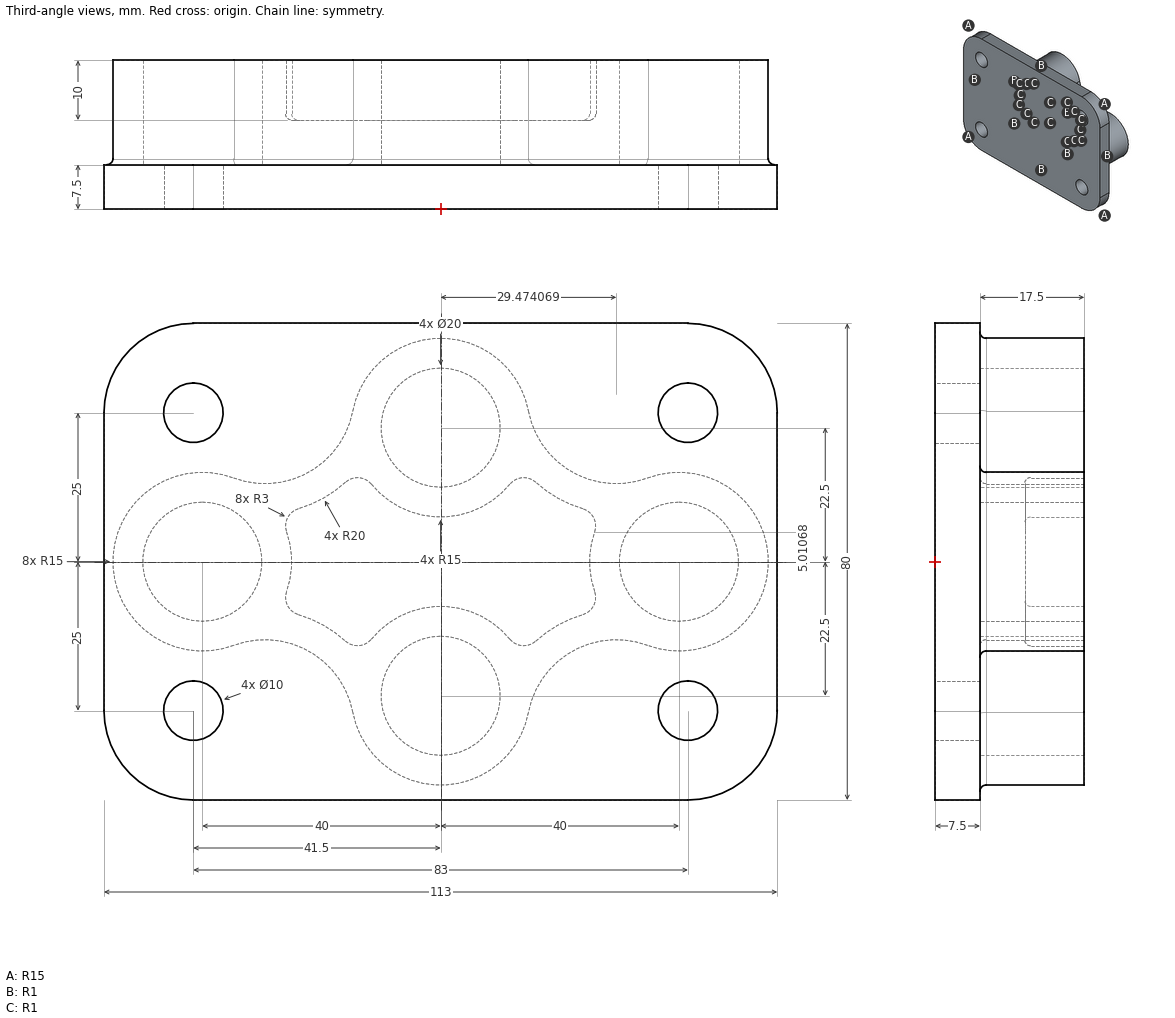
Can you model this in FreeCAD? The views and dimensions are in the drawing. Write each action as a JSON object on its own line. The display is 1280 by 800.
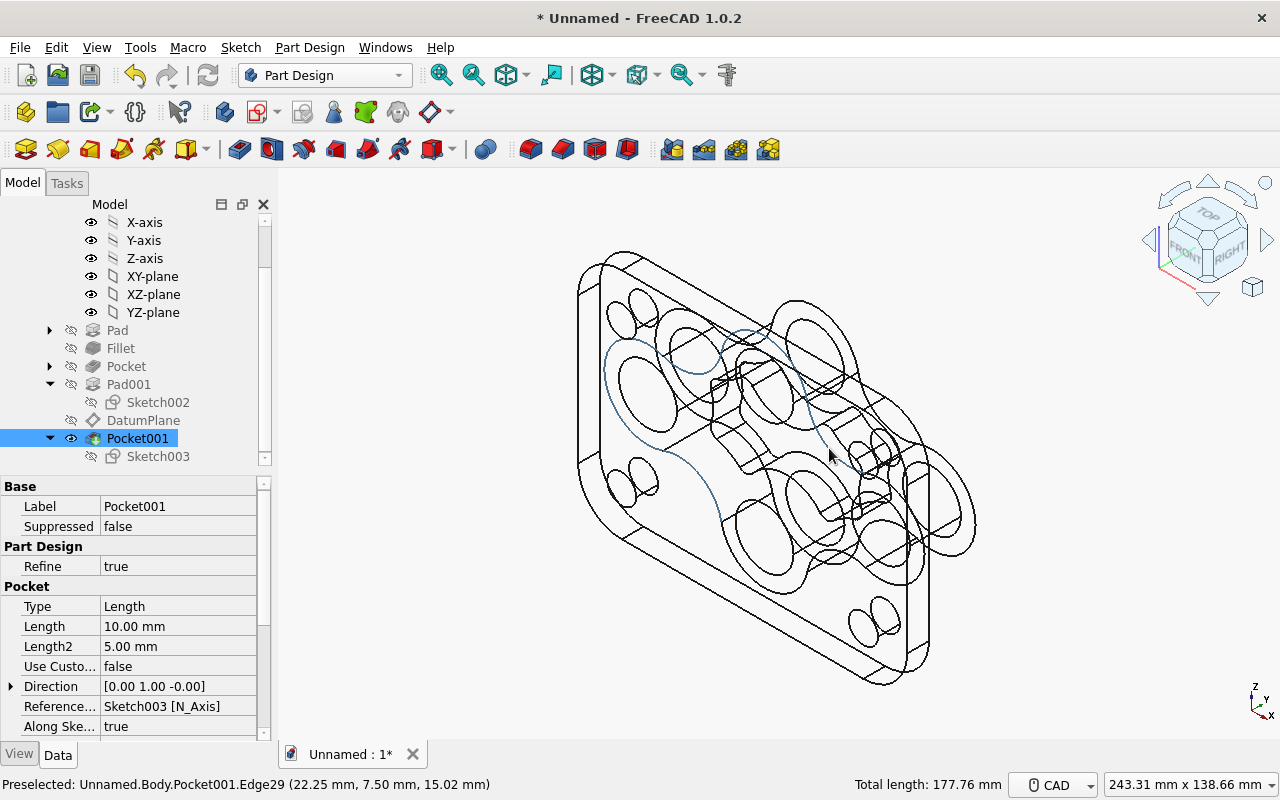
{"action": "left_click", "coordinate": [921, 533], "text": "ctrl"}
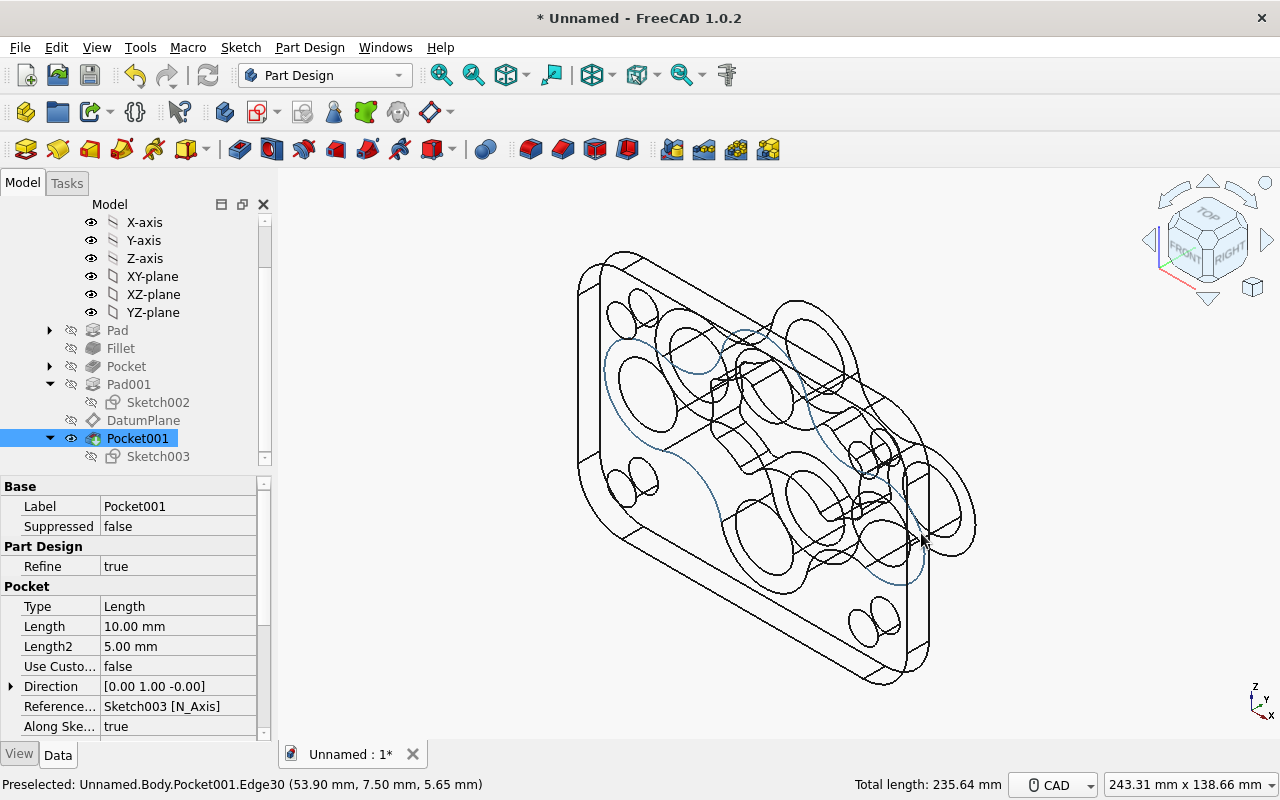
{"action": "left_click", "coordinate": [829, 549], "text": "ctrl"}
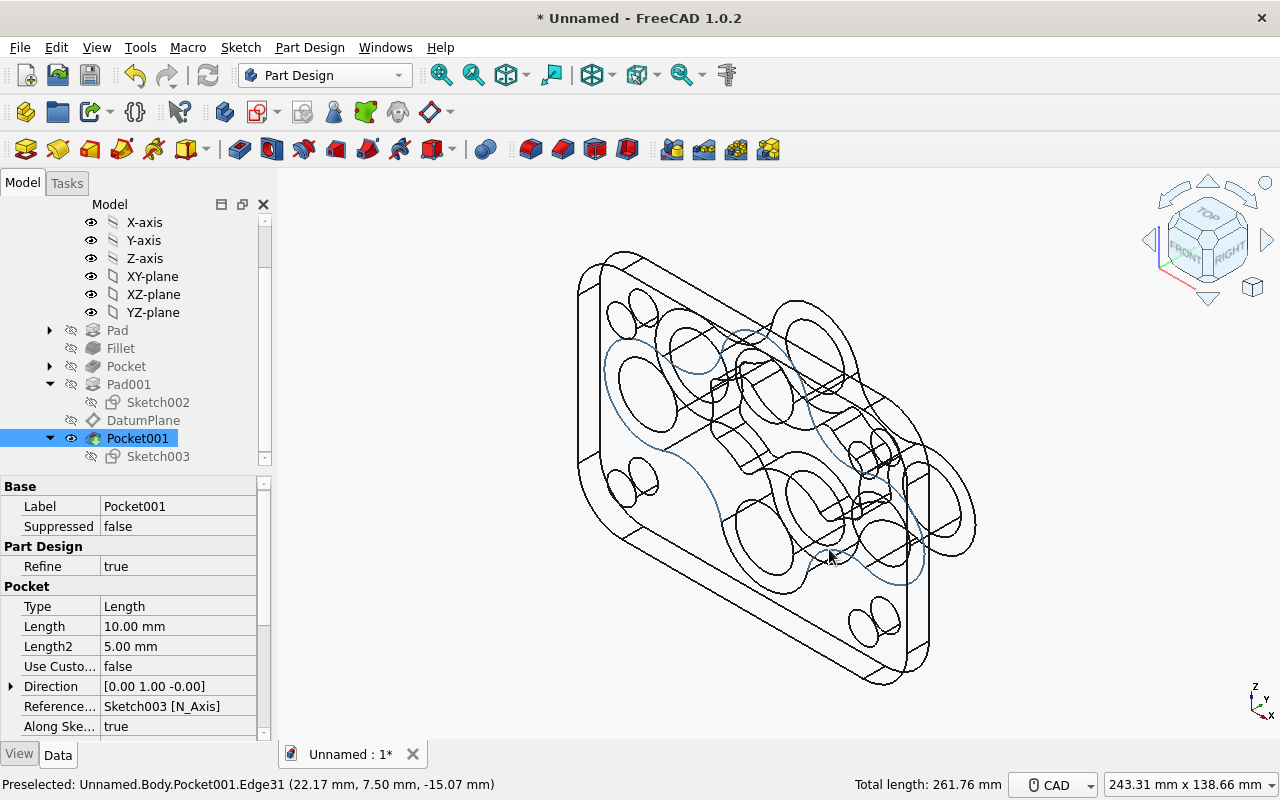
{"action": "left_click", "coordinate": [764, 587], "text": "ctrl"}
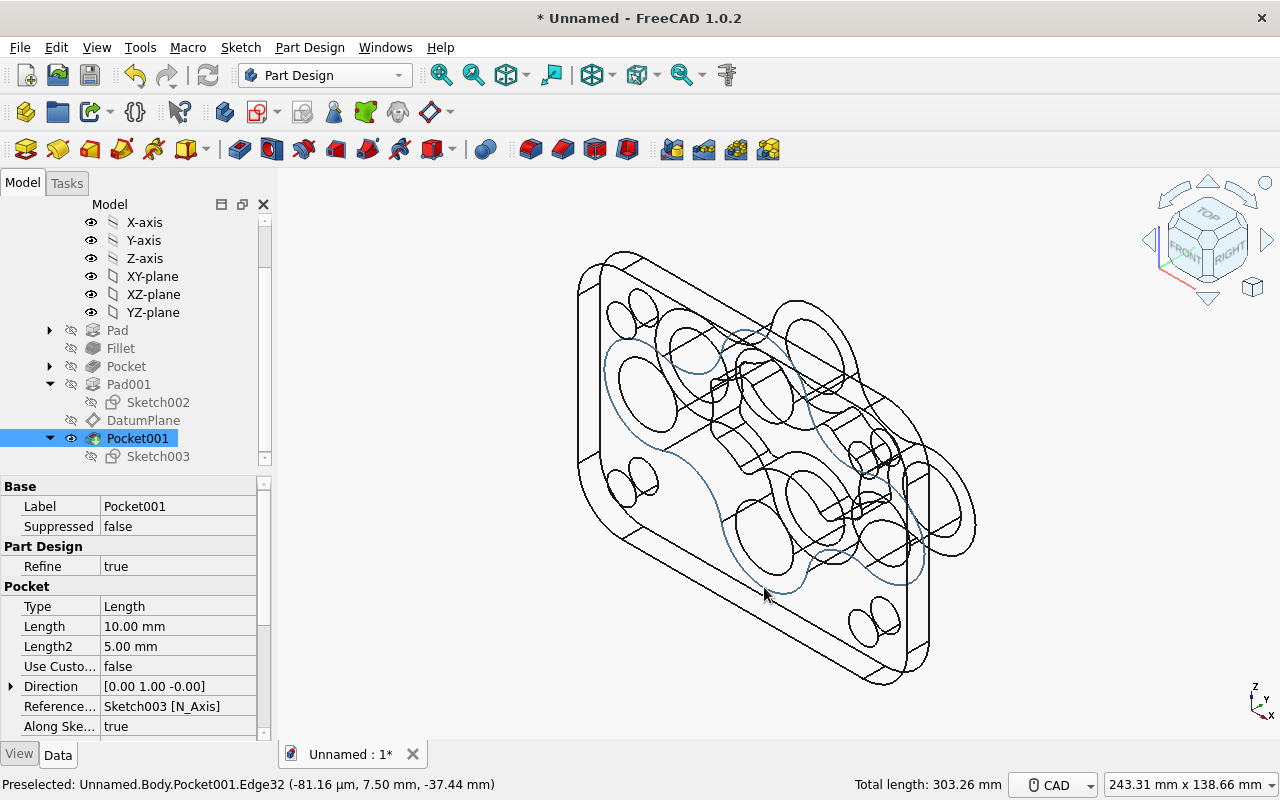
{"action": "key", "text": "v 1"}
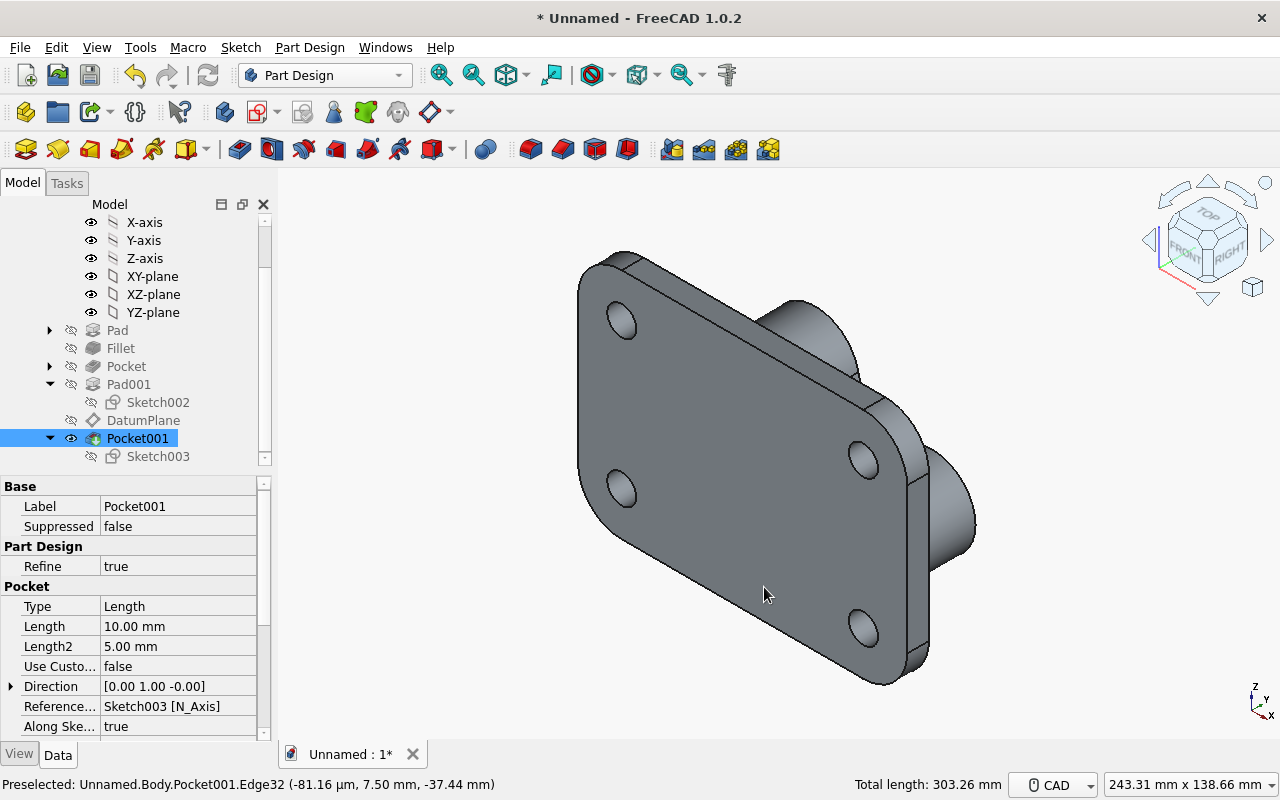
{"action": "left_click", "coordinate": [532, 150]}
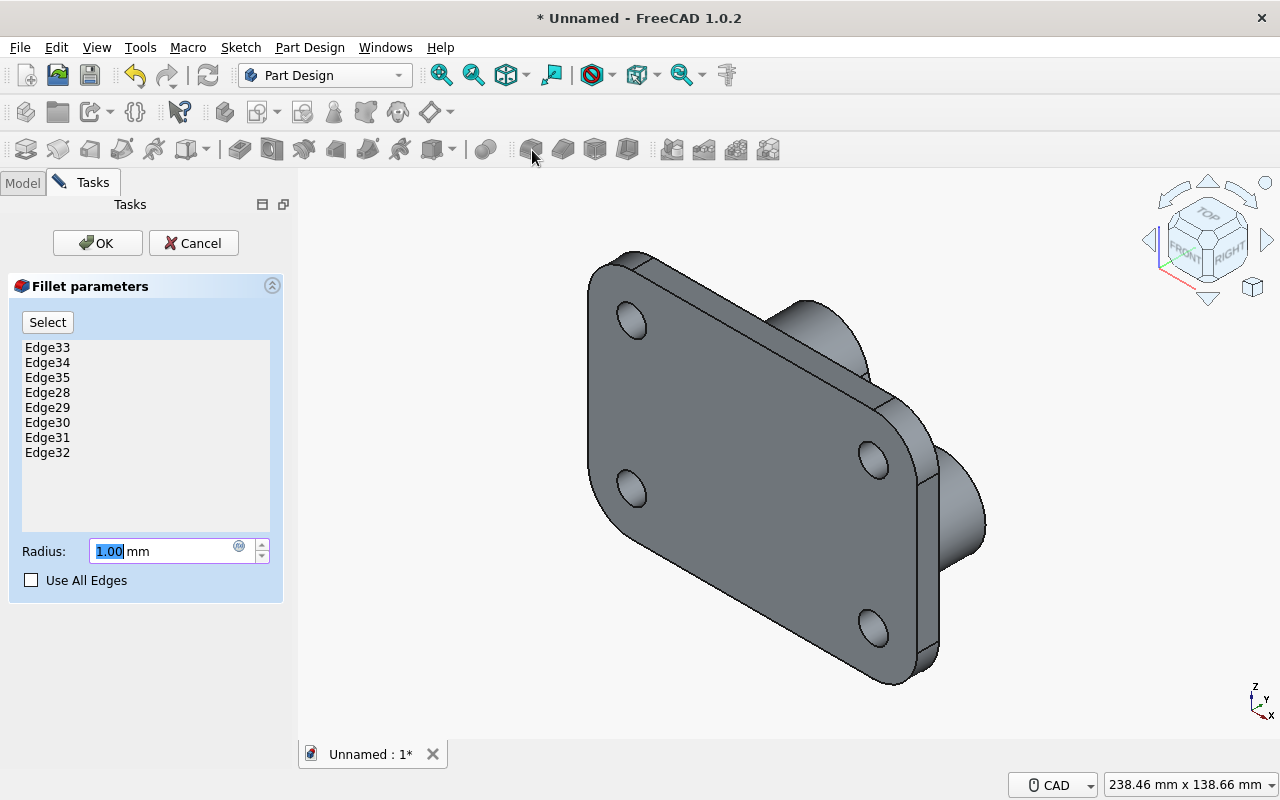
{"action": "type", "text": "1"}
{"action": "key", "text": "Tab"}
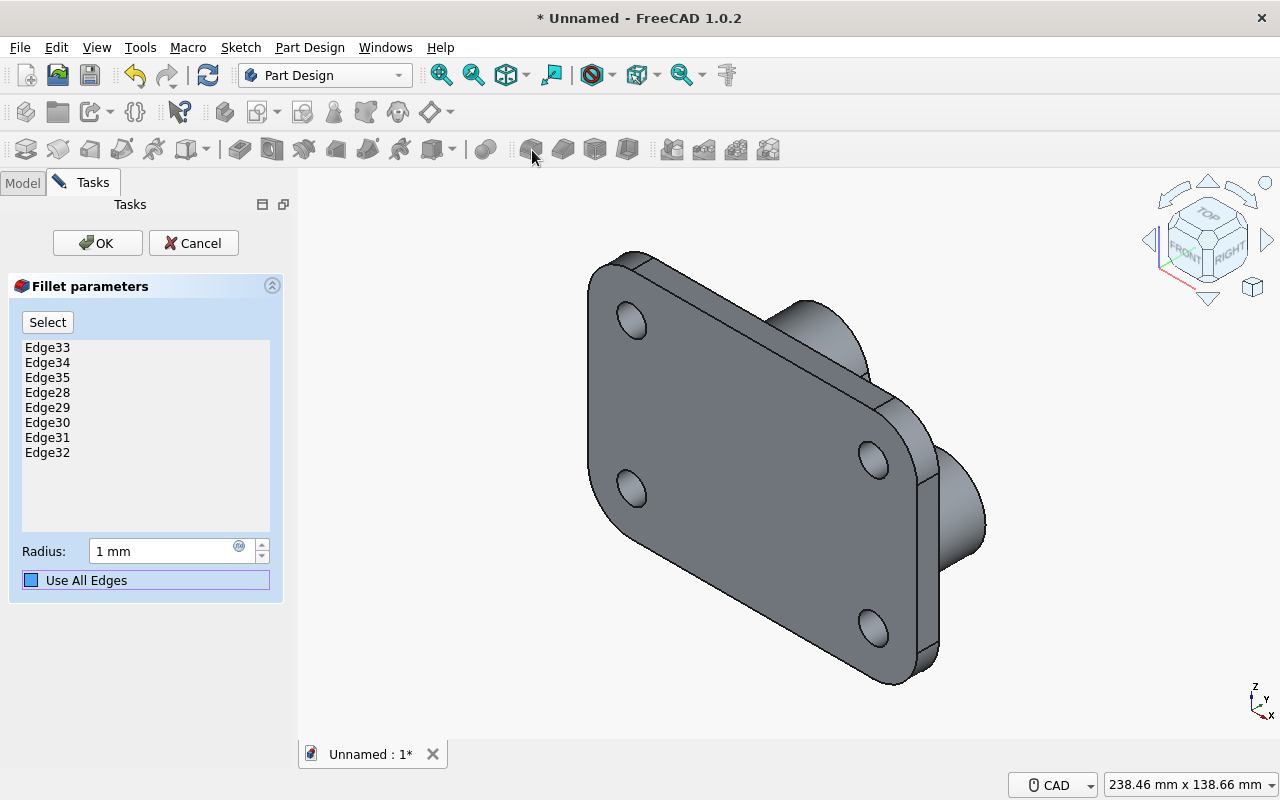
{"action": "left_click", "coordinate": [98, 243]}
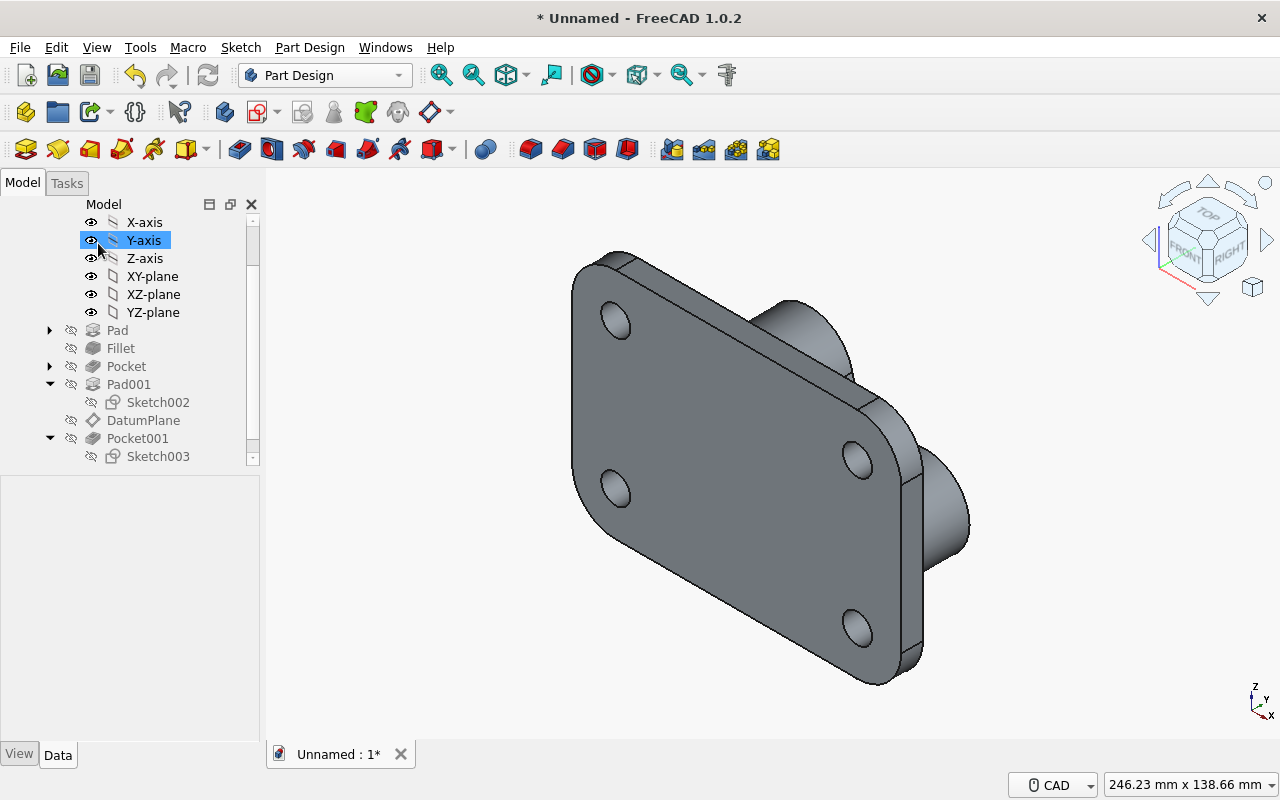
{"action": "key", "text": "2"}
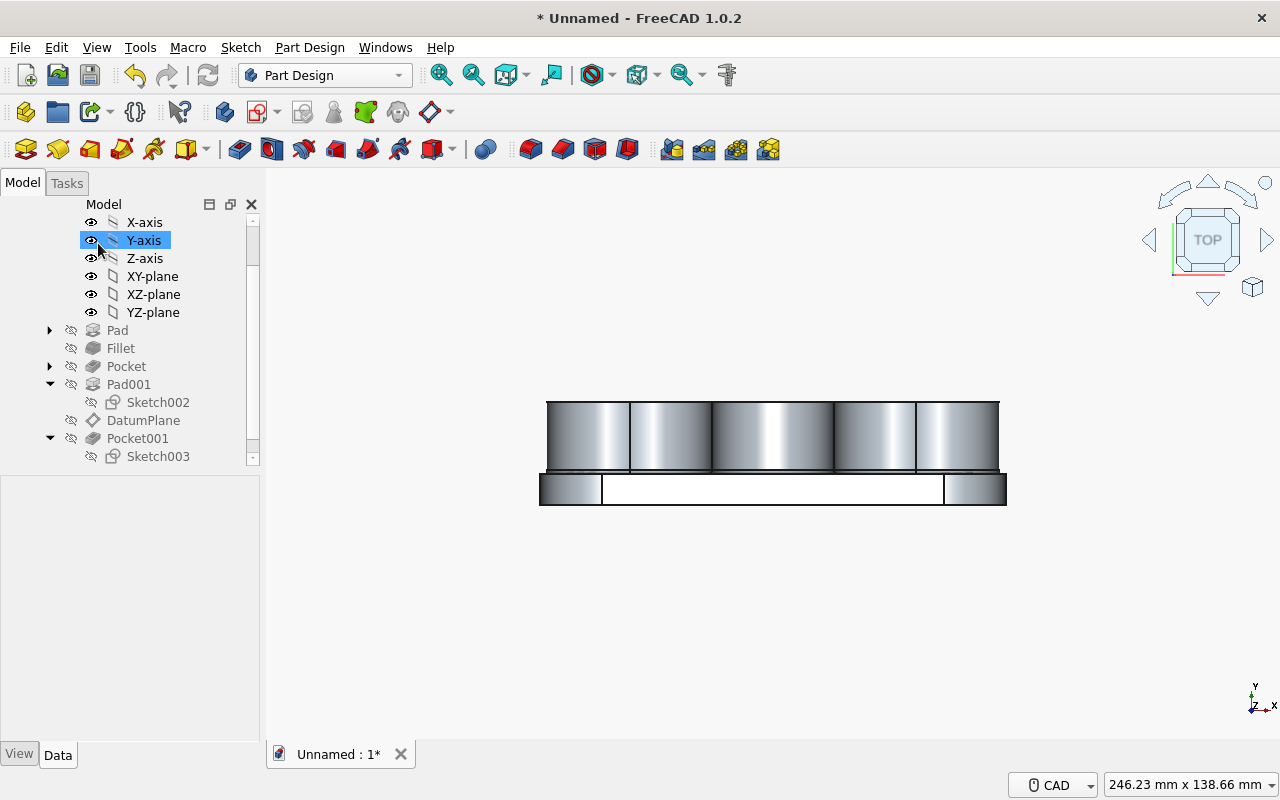
{"action": "key", "text": "0"}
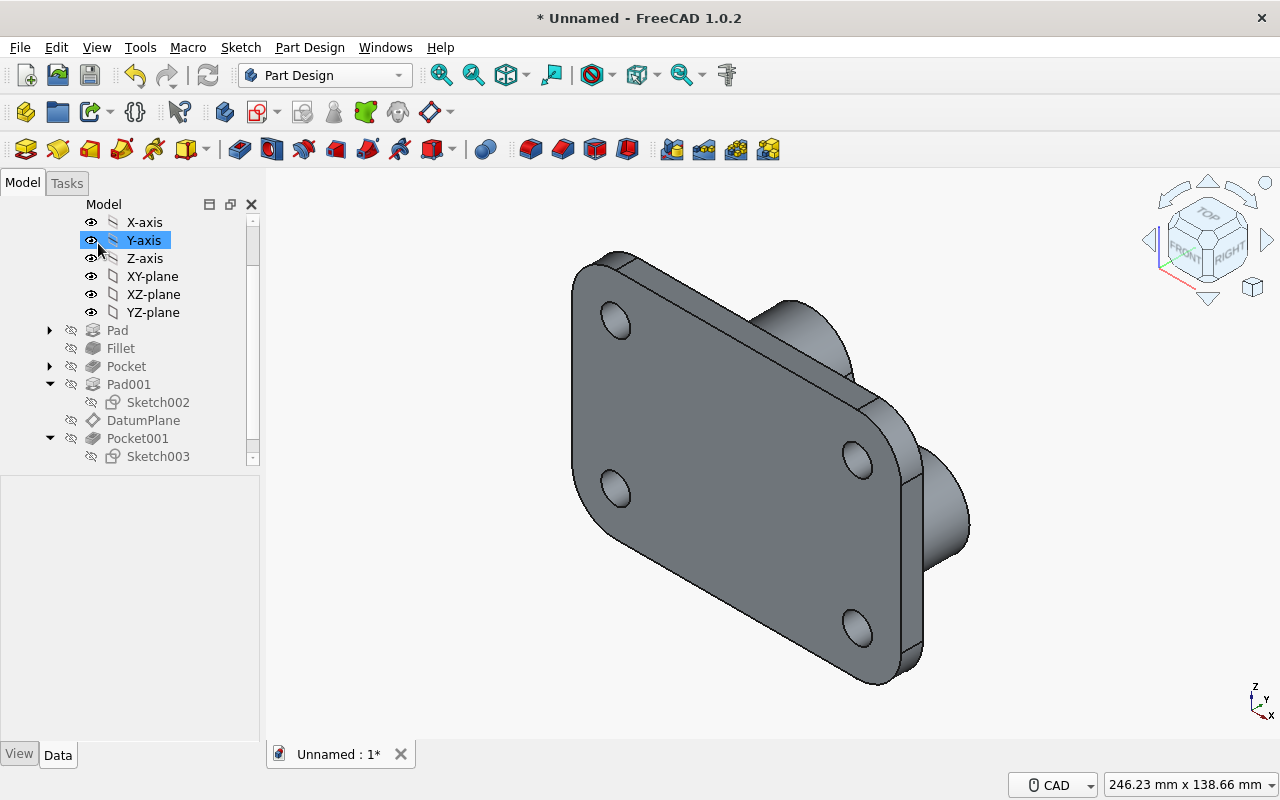
{"action": "key", "text": "1"}